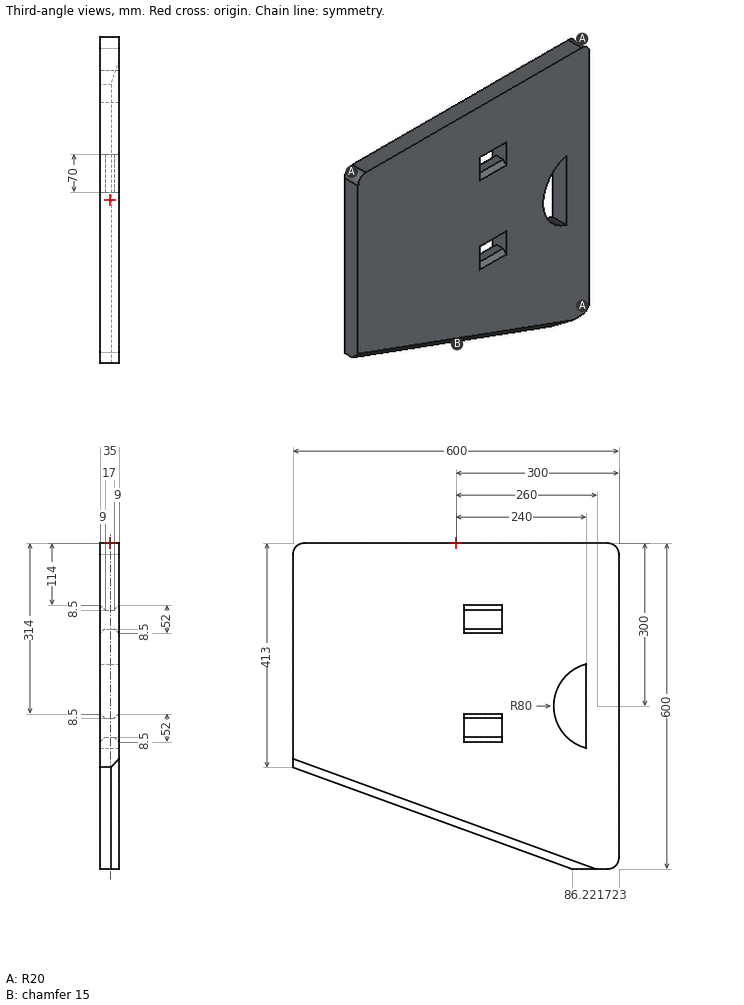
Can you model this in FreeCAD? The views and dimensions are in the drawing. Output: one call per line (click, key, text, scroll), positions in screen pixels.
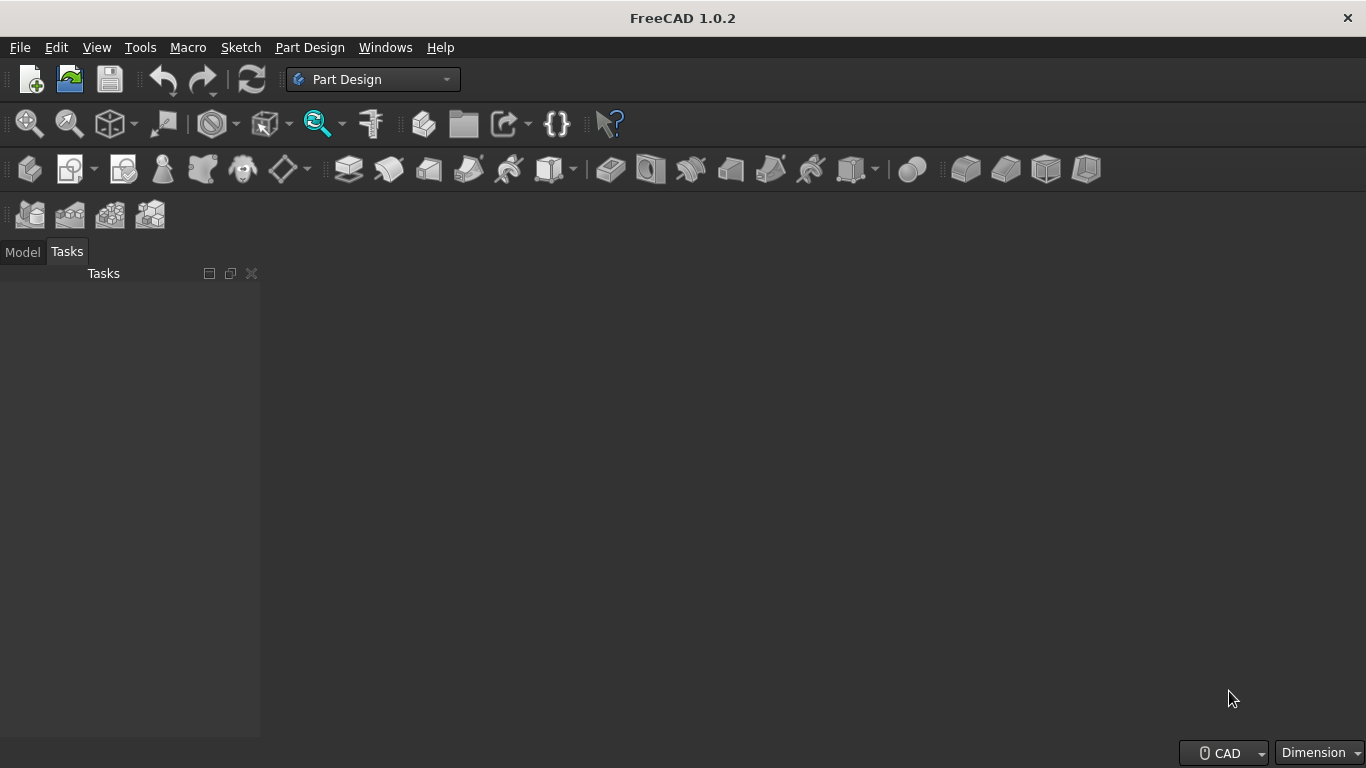
key(ctrl+n)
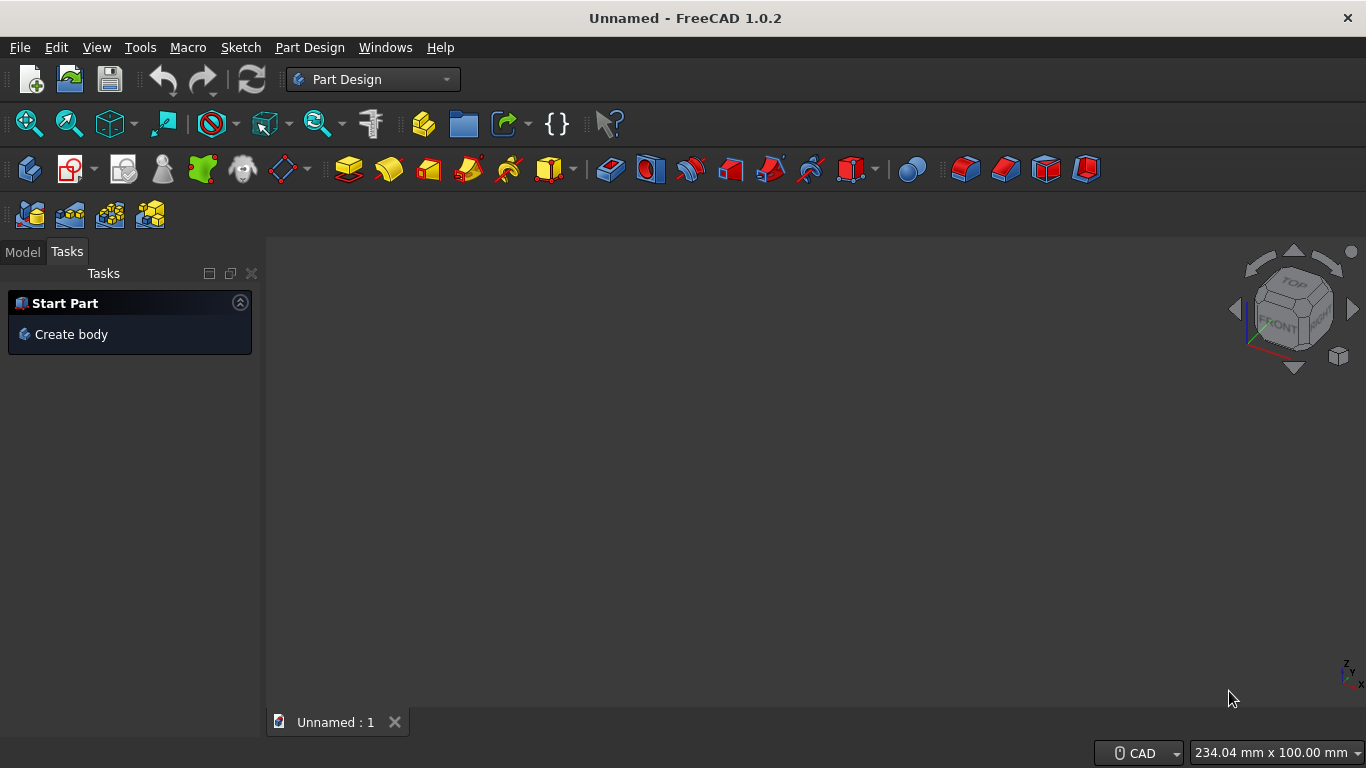
click(70, 170)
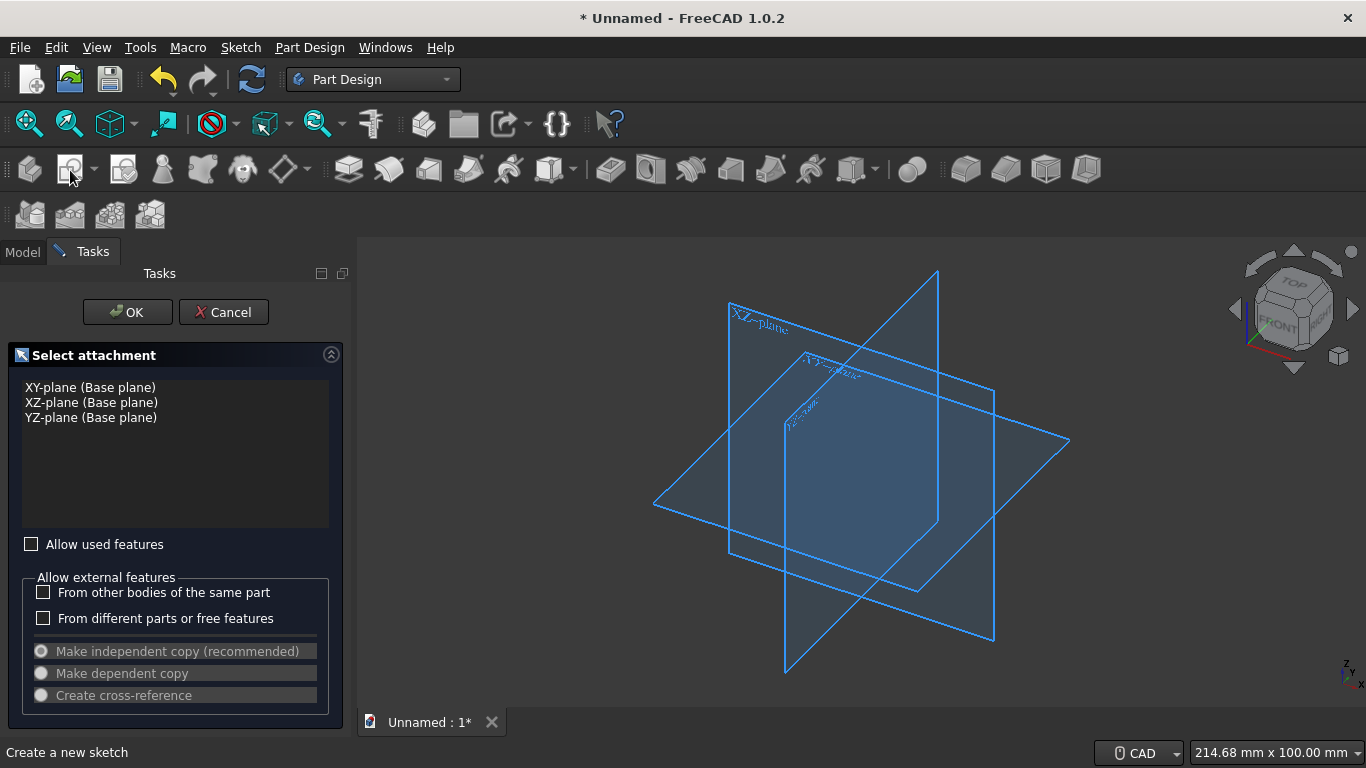
click(82, 418)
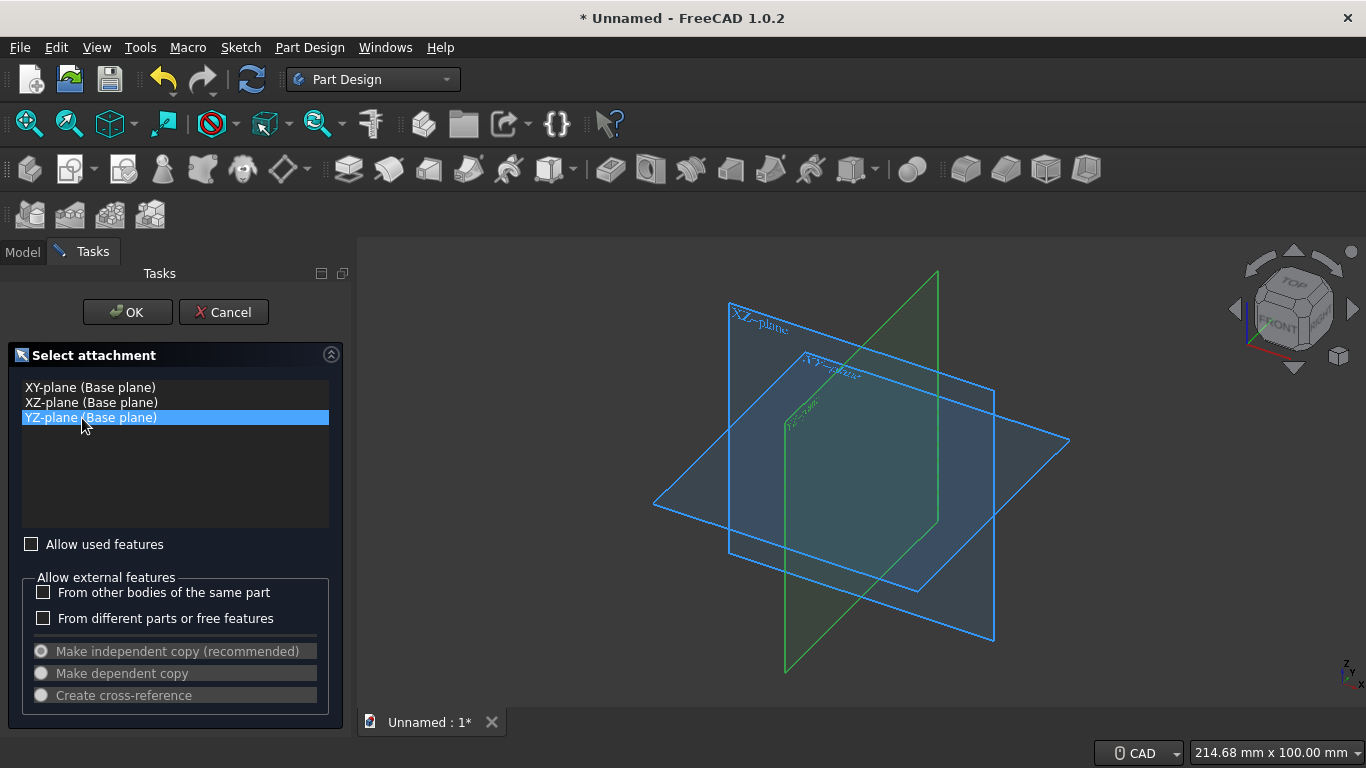
click(128, 312)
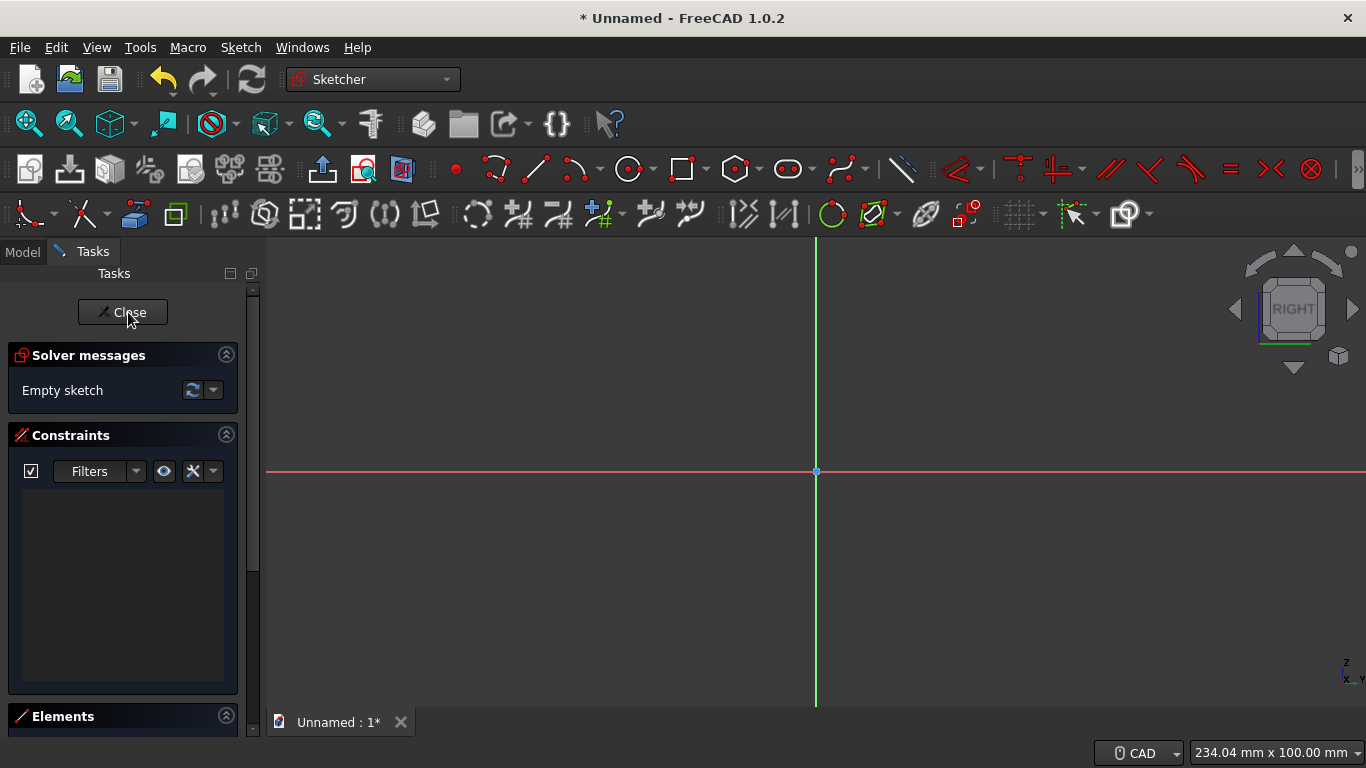
scroll(739, 296, down, 11)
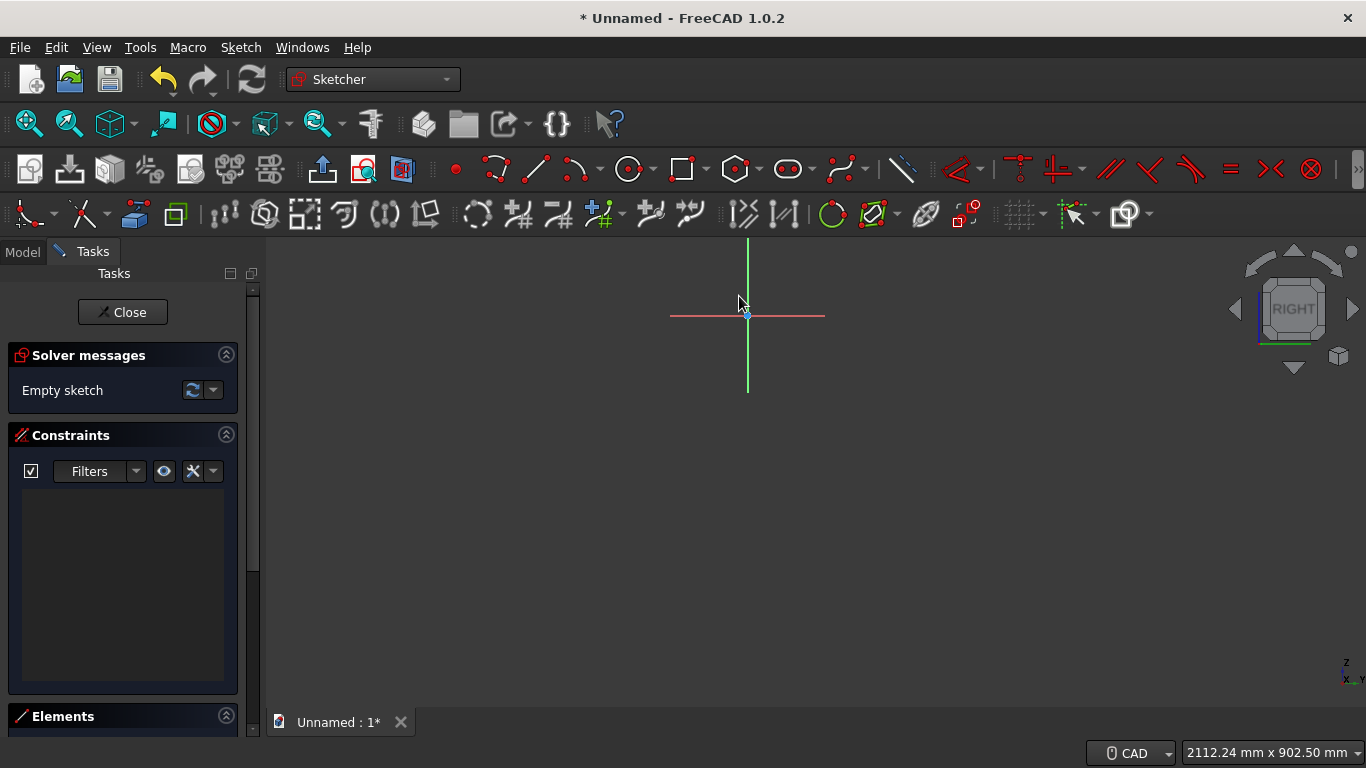
click(496, 170)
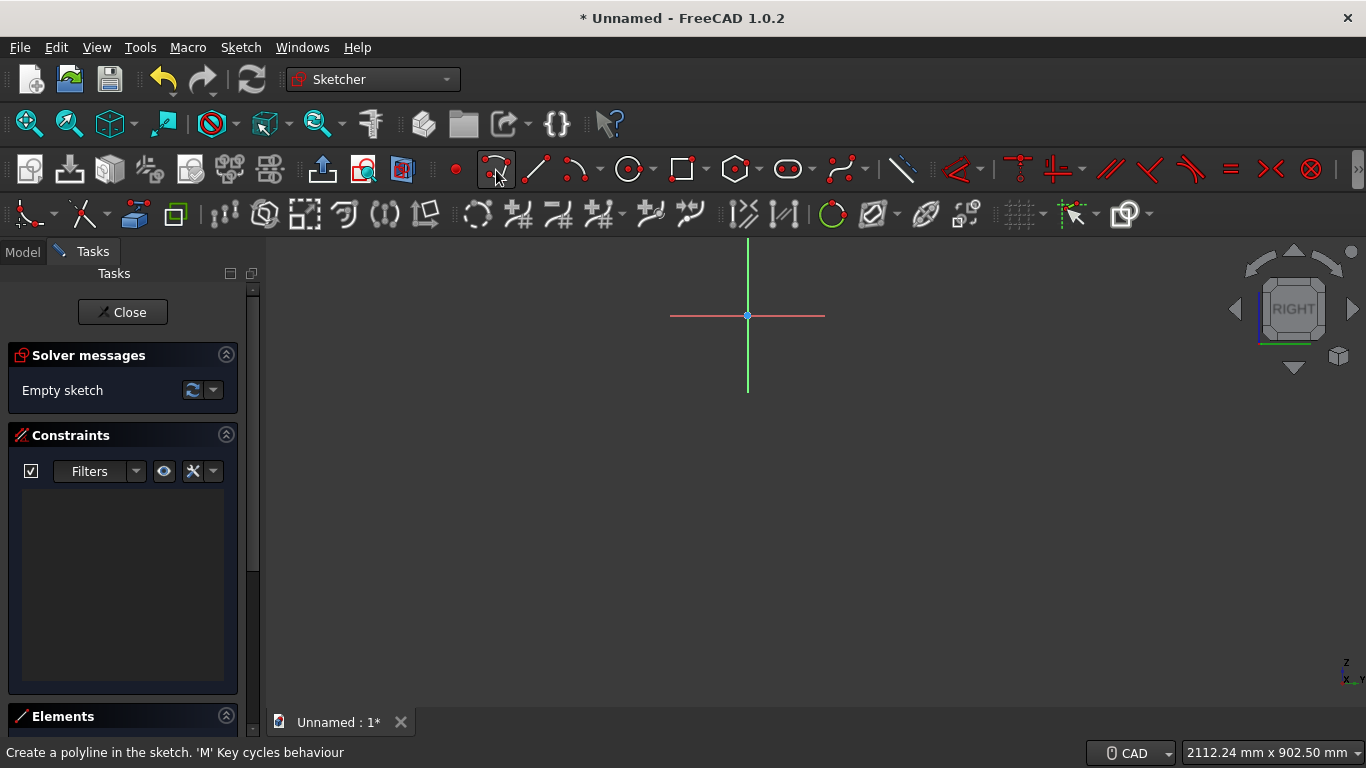
click(904, 316)
click(592, 325)
click(592, 531)
click(859, 628)
click(904, 628)
click(904, 317)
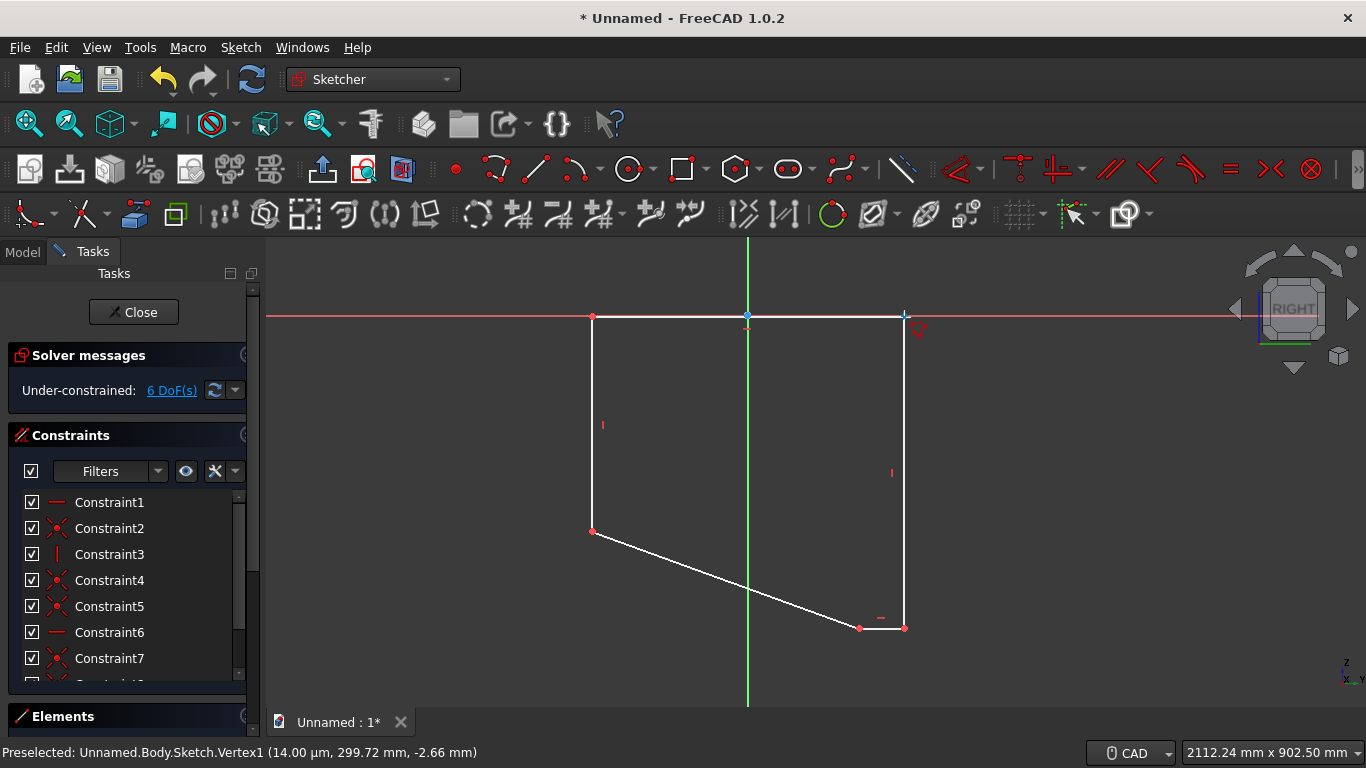
click(536, 170)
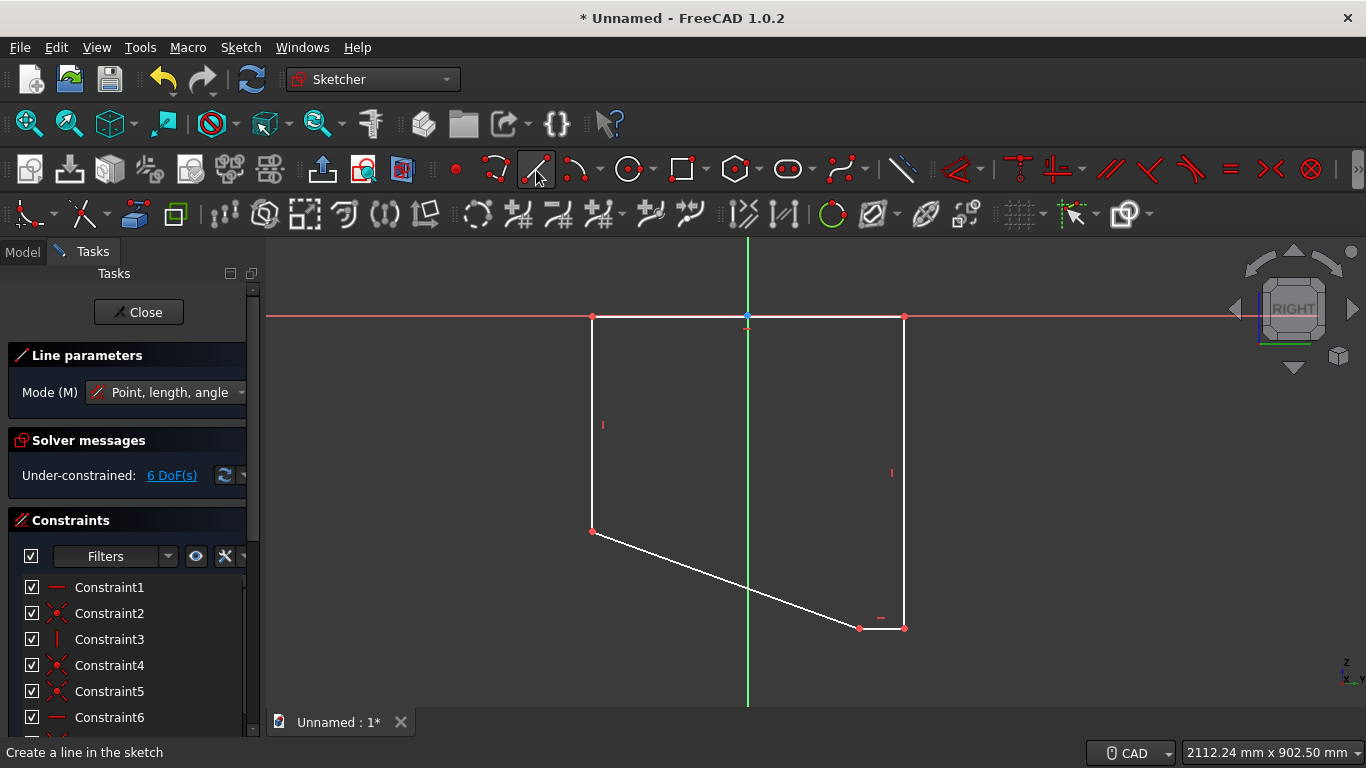
click(873, 432)
click(873, 512)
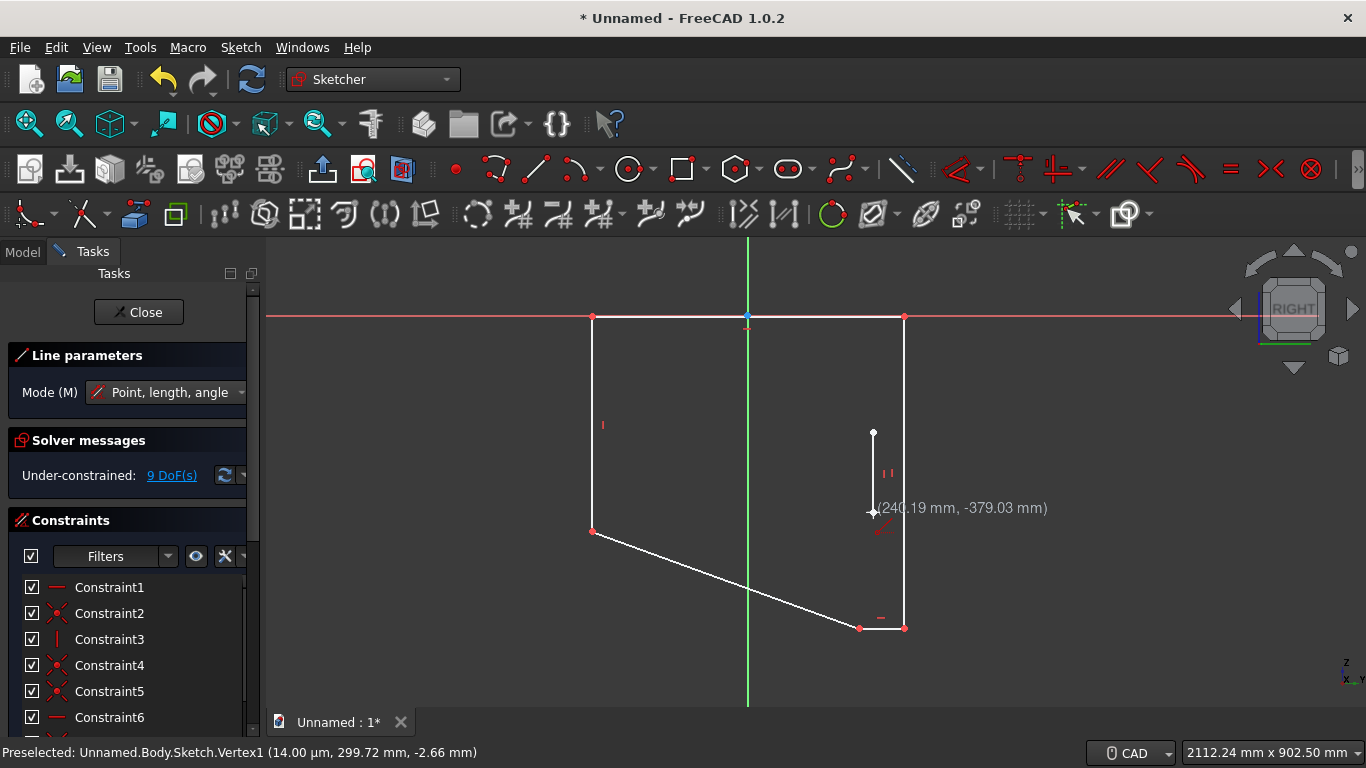
key(g)
key(3)
key(a)